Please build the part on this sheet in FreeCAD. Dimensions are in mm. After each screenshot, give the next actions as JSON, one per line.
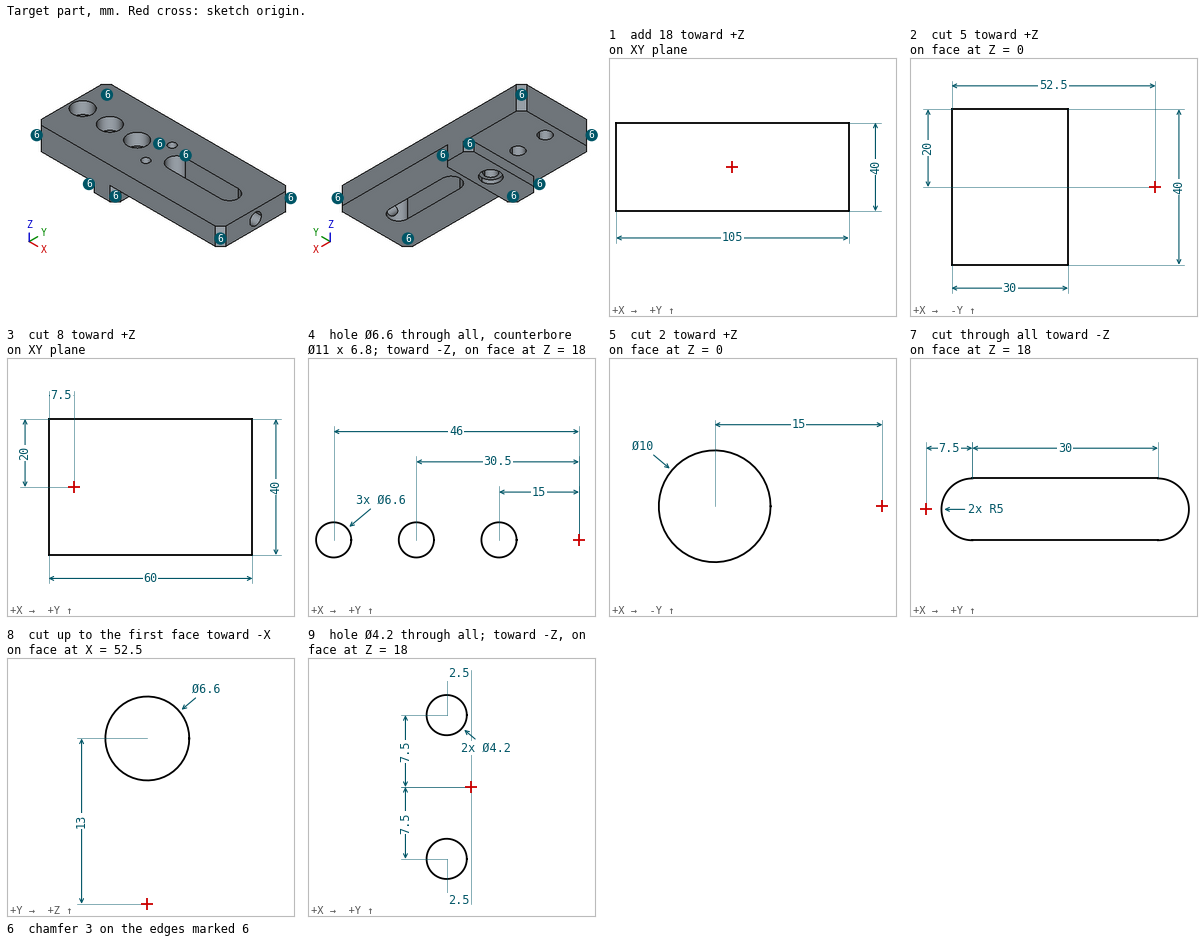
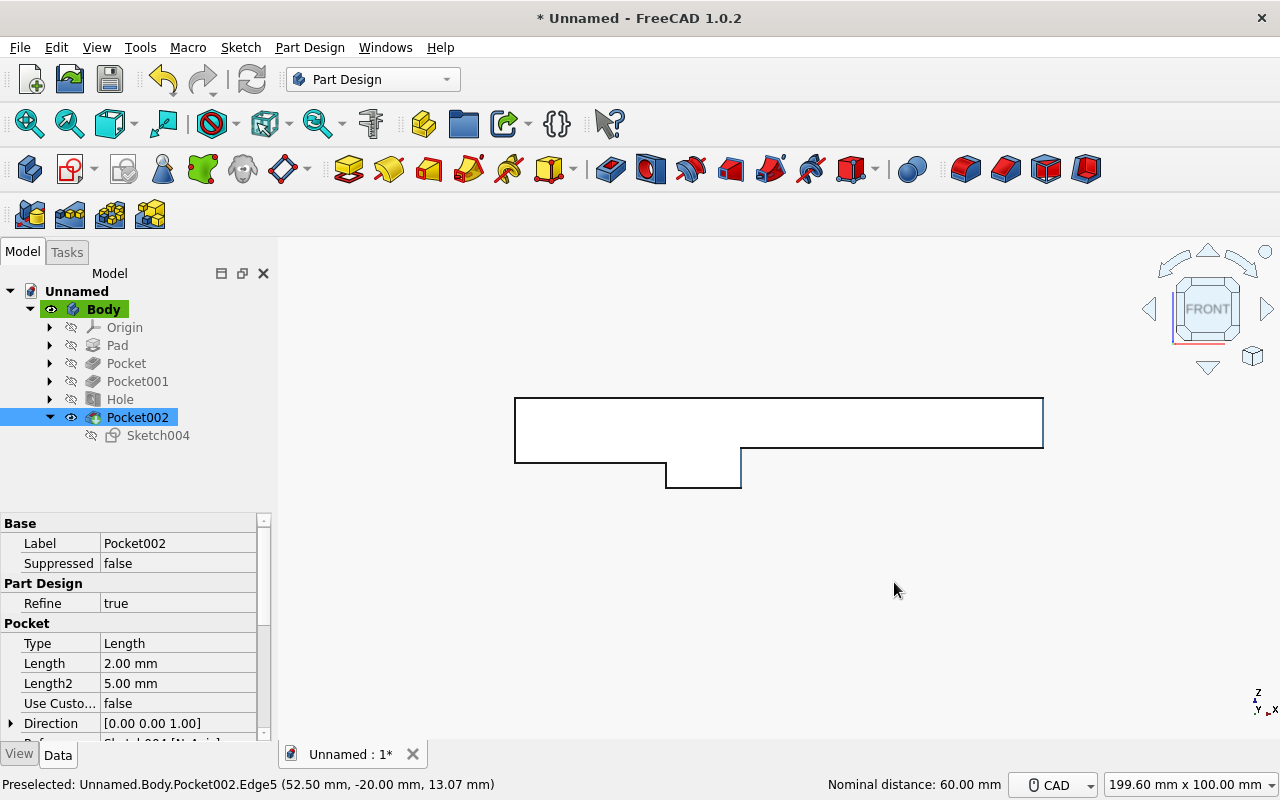
{"action": "left_click", "coordinate": [666, 474], "text": "ctrl"}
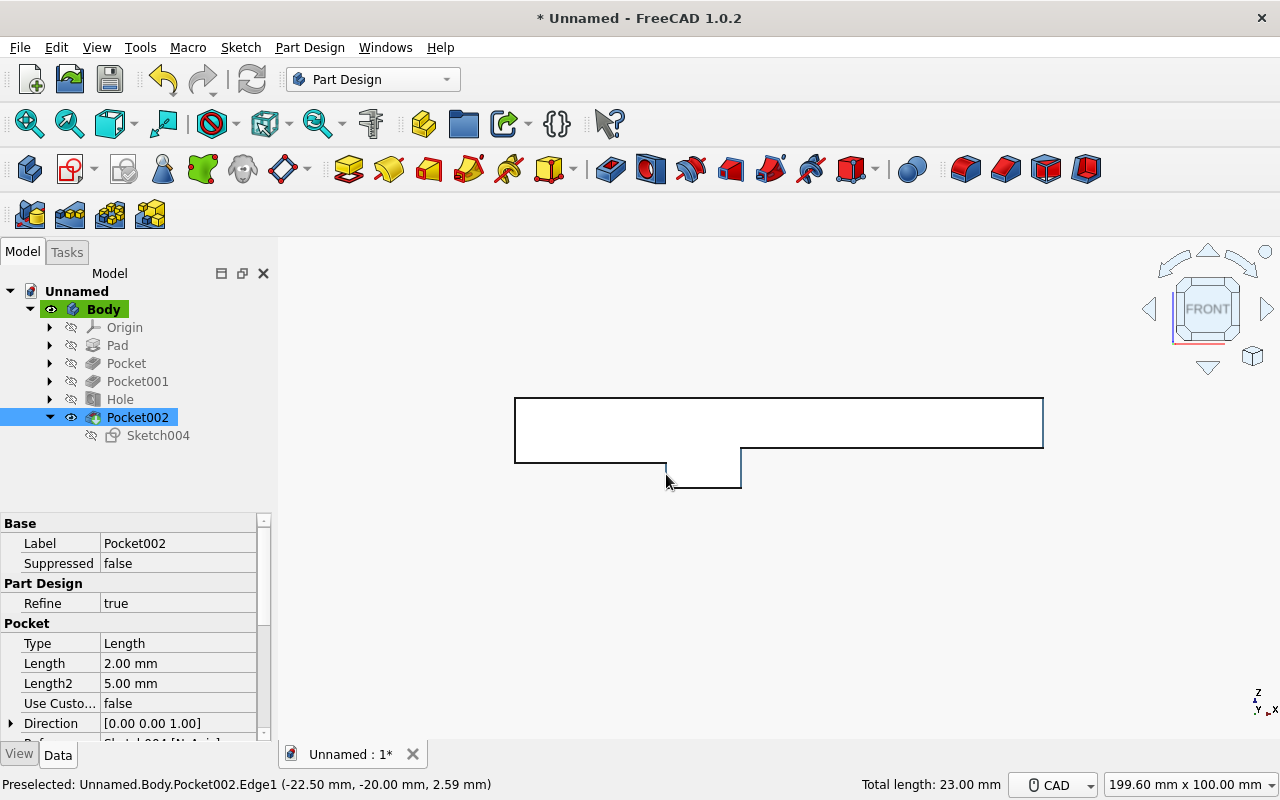
{"action": "left_click", "coordinate": [515, 429], "text": "ctrl"}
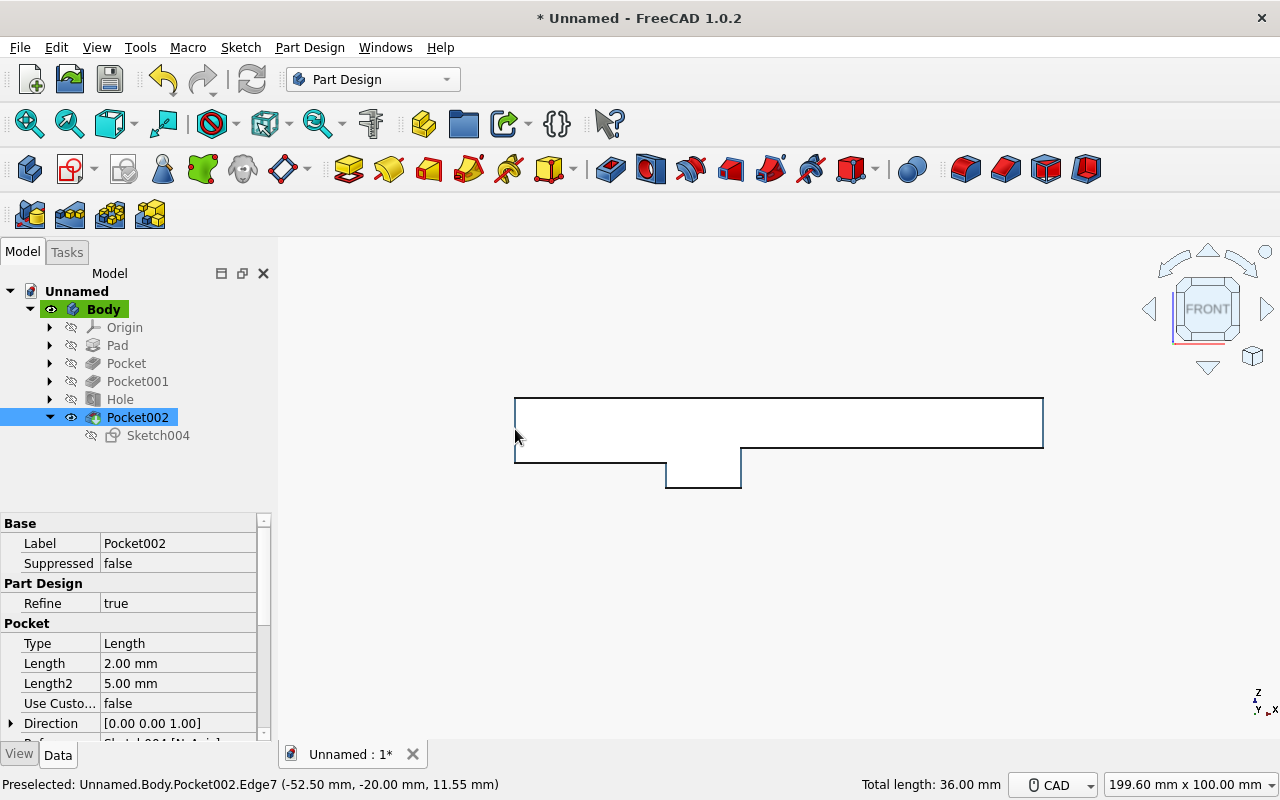
{"action": "key", "text": "3"}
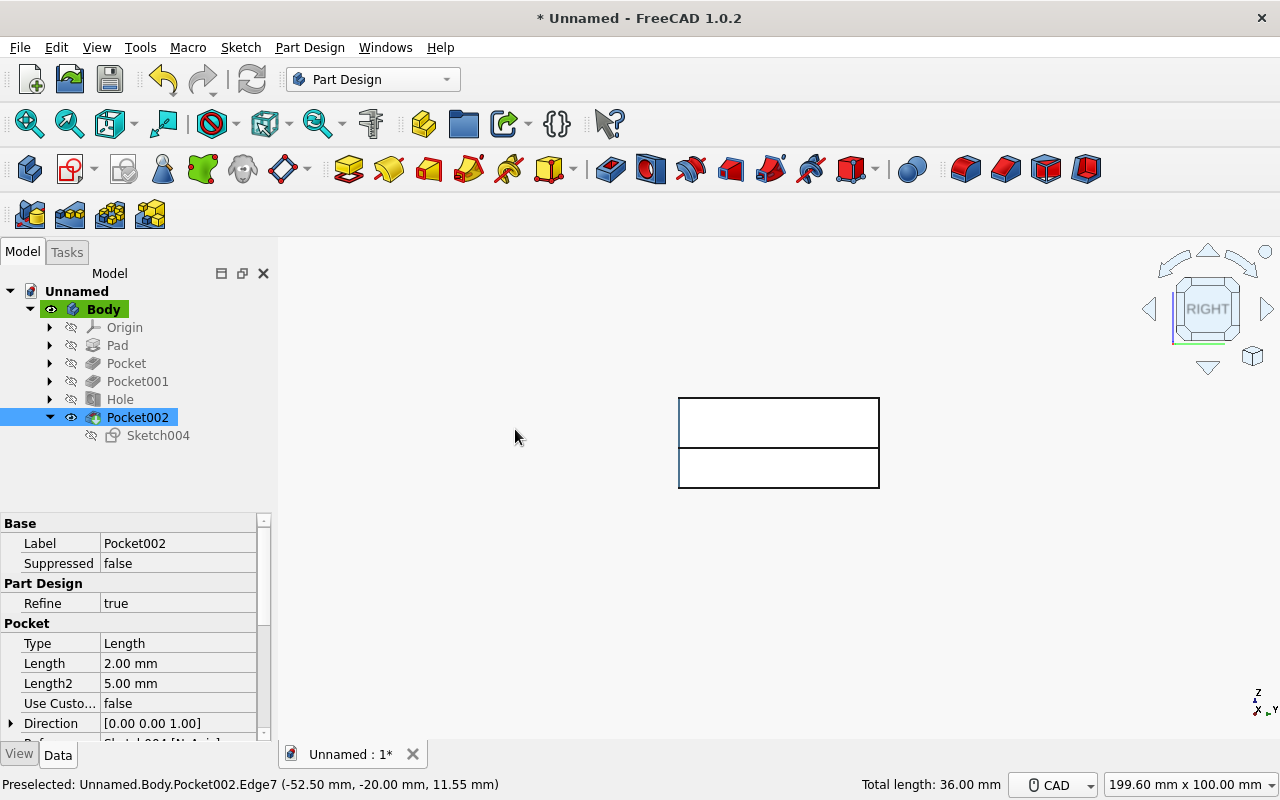
{"action": "key", "text": "v f"}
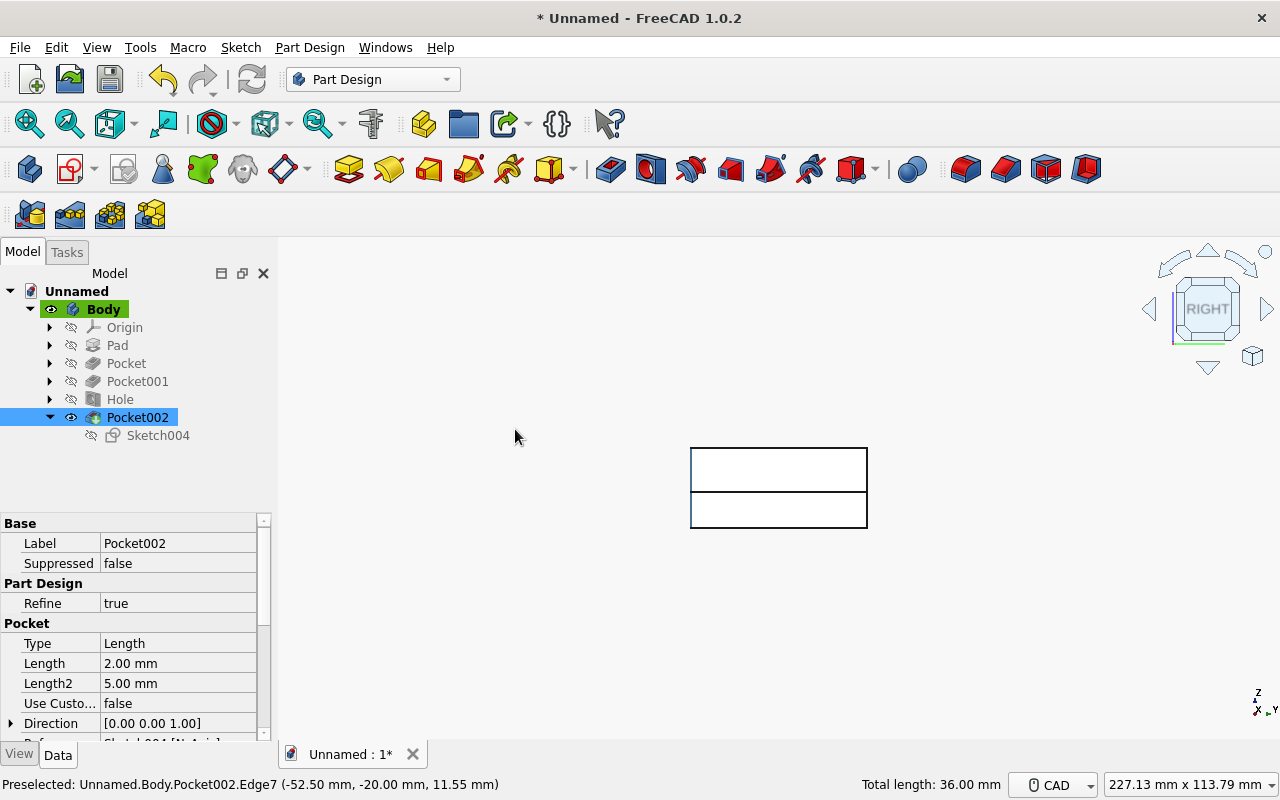
{"action": "left_click", "coordinate": [867, 509], "text": "ctrl"}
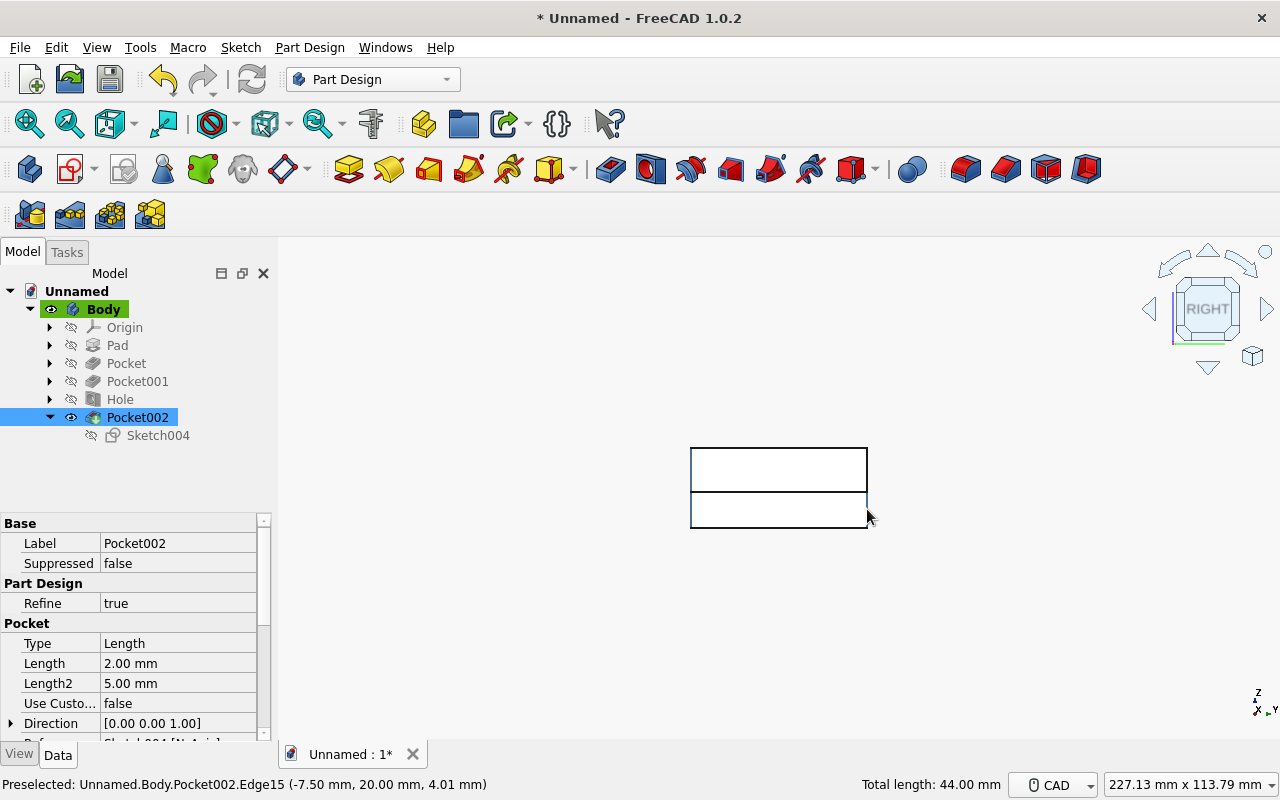
{"action": "left_click", "coordinate": [867, 469], "text": "ctrl"}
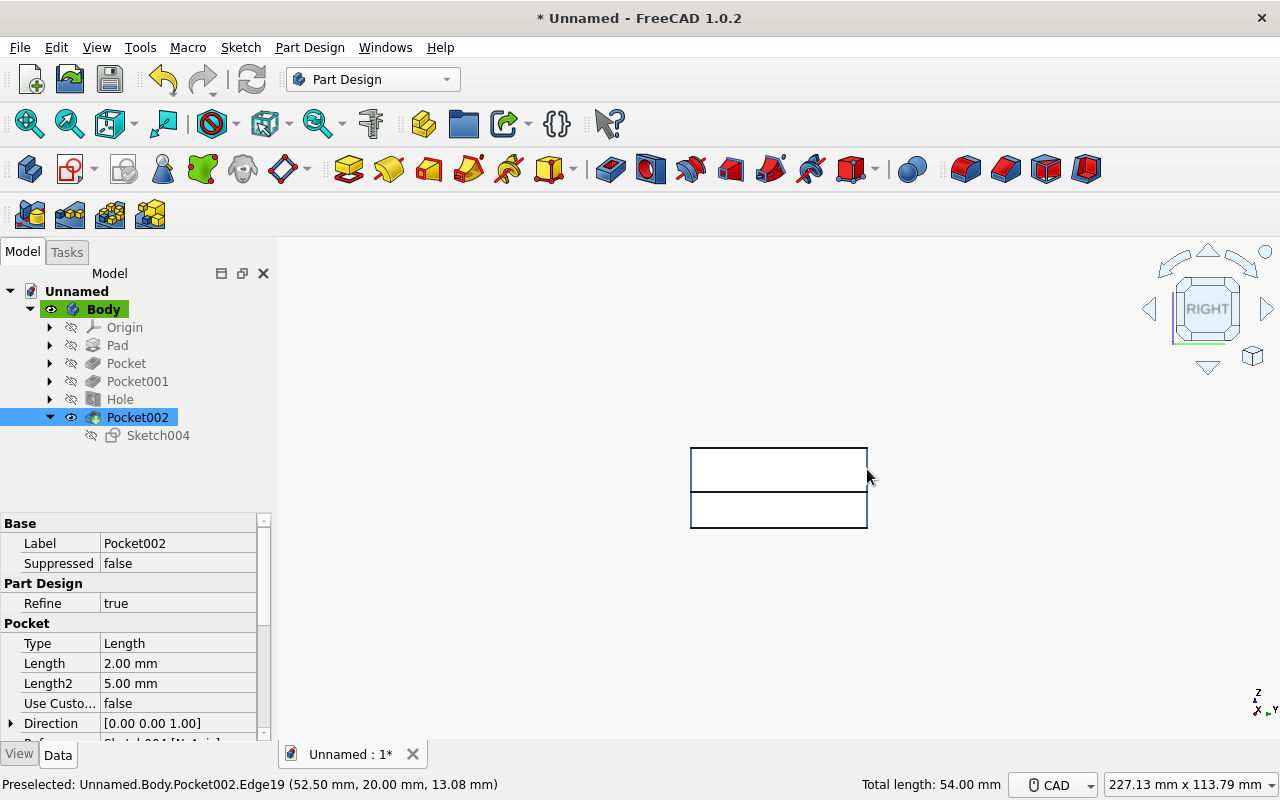
{"action": "key", "text": "5"}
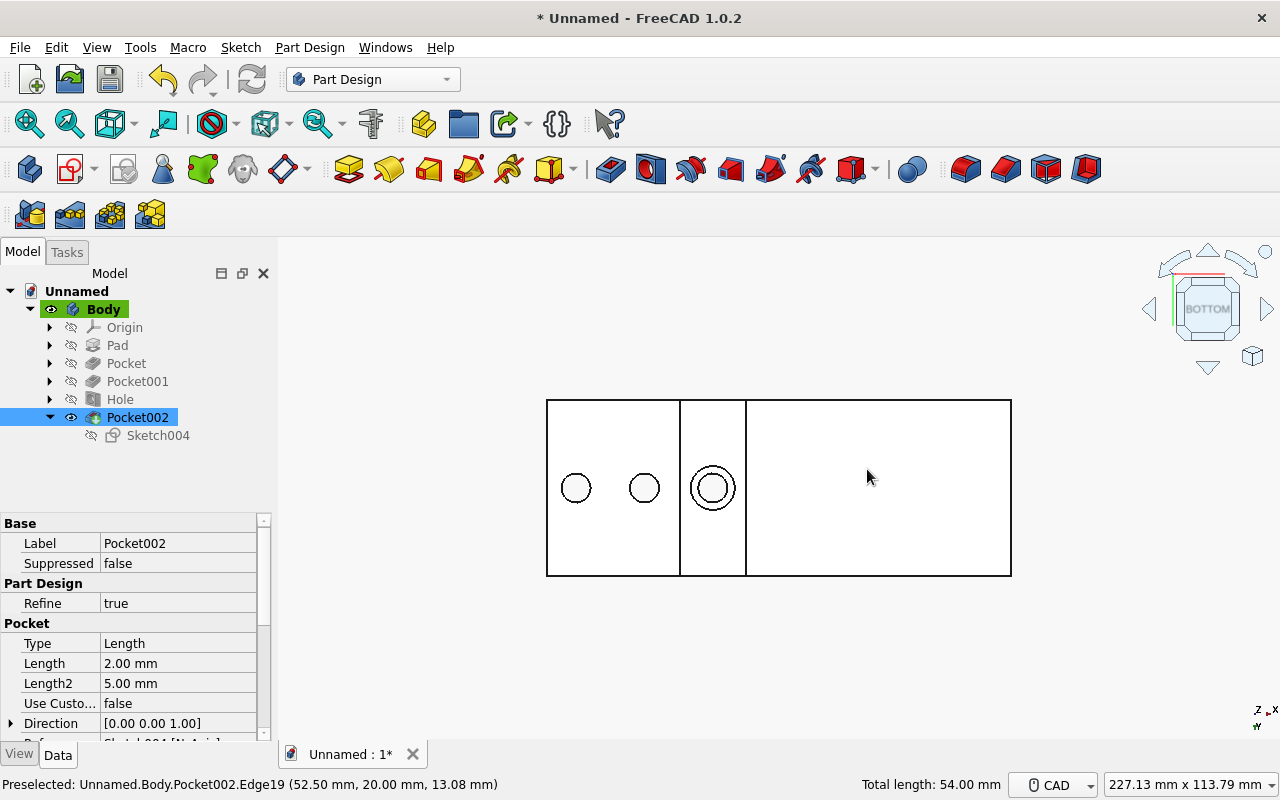
{"action": "key", "text": "4"}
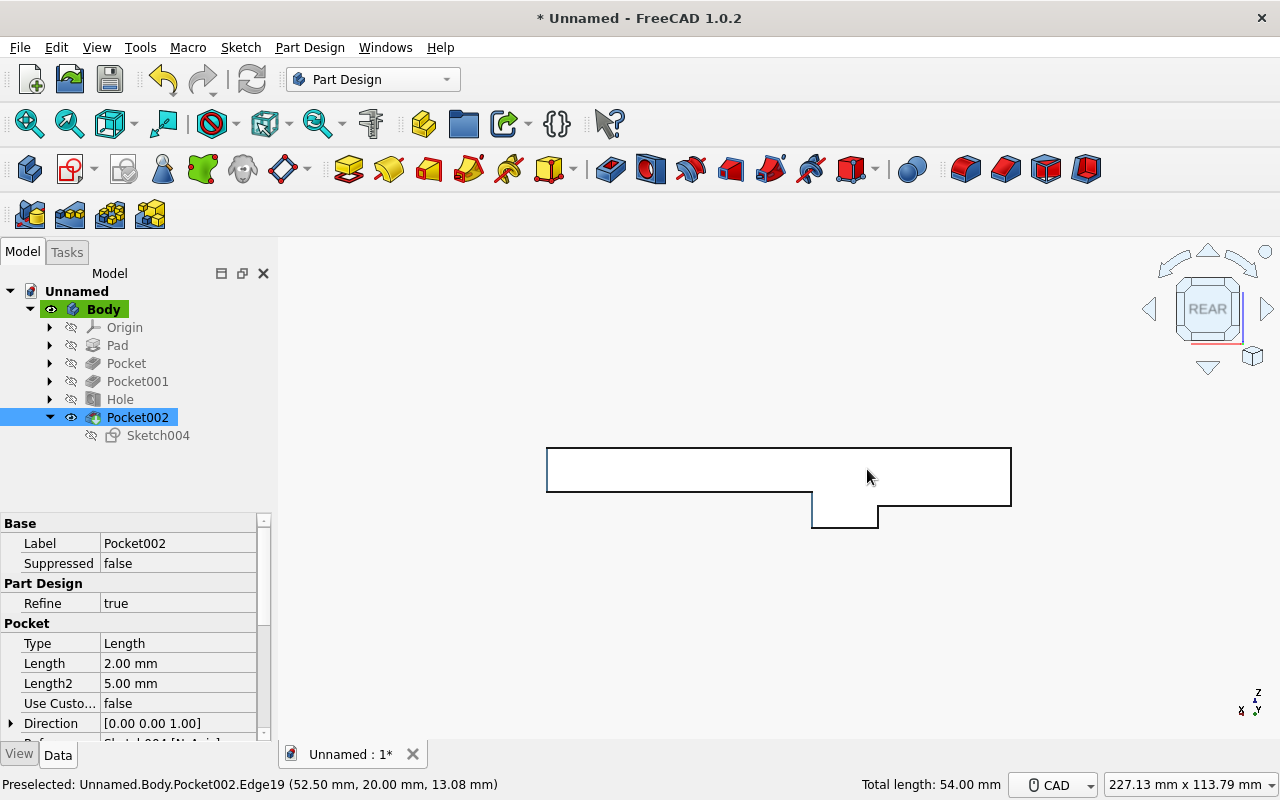
{"action": "left_click", "coordinate": [878, 516], "text": "ctrl"}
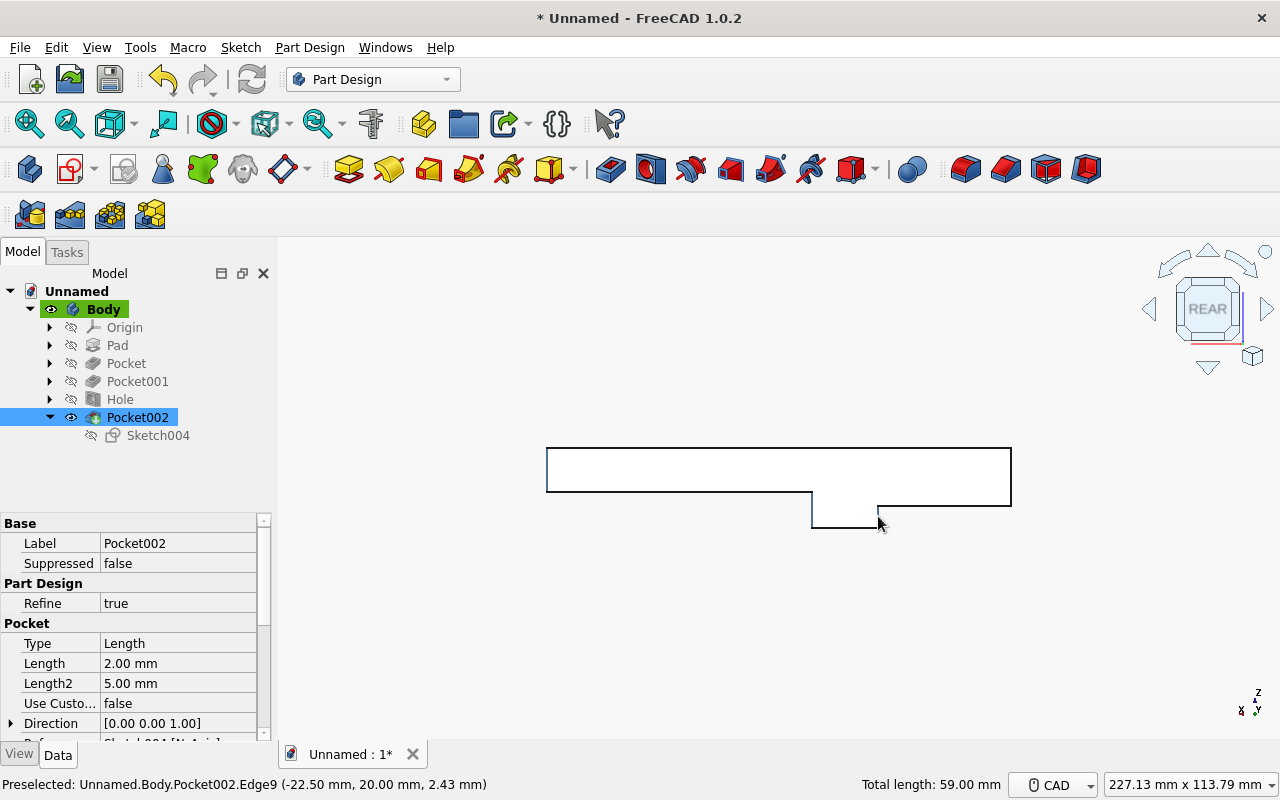
{"action": "left_click", "coordinate": [1011, 476], "text": "ctrl"}